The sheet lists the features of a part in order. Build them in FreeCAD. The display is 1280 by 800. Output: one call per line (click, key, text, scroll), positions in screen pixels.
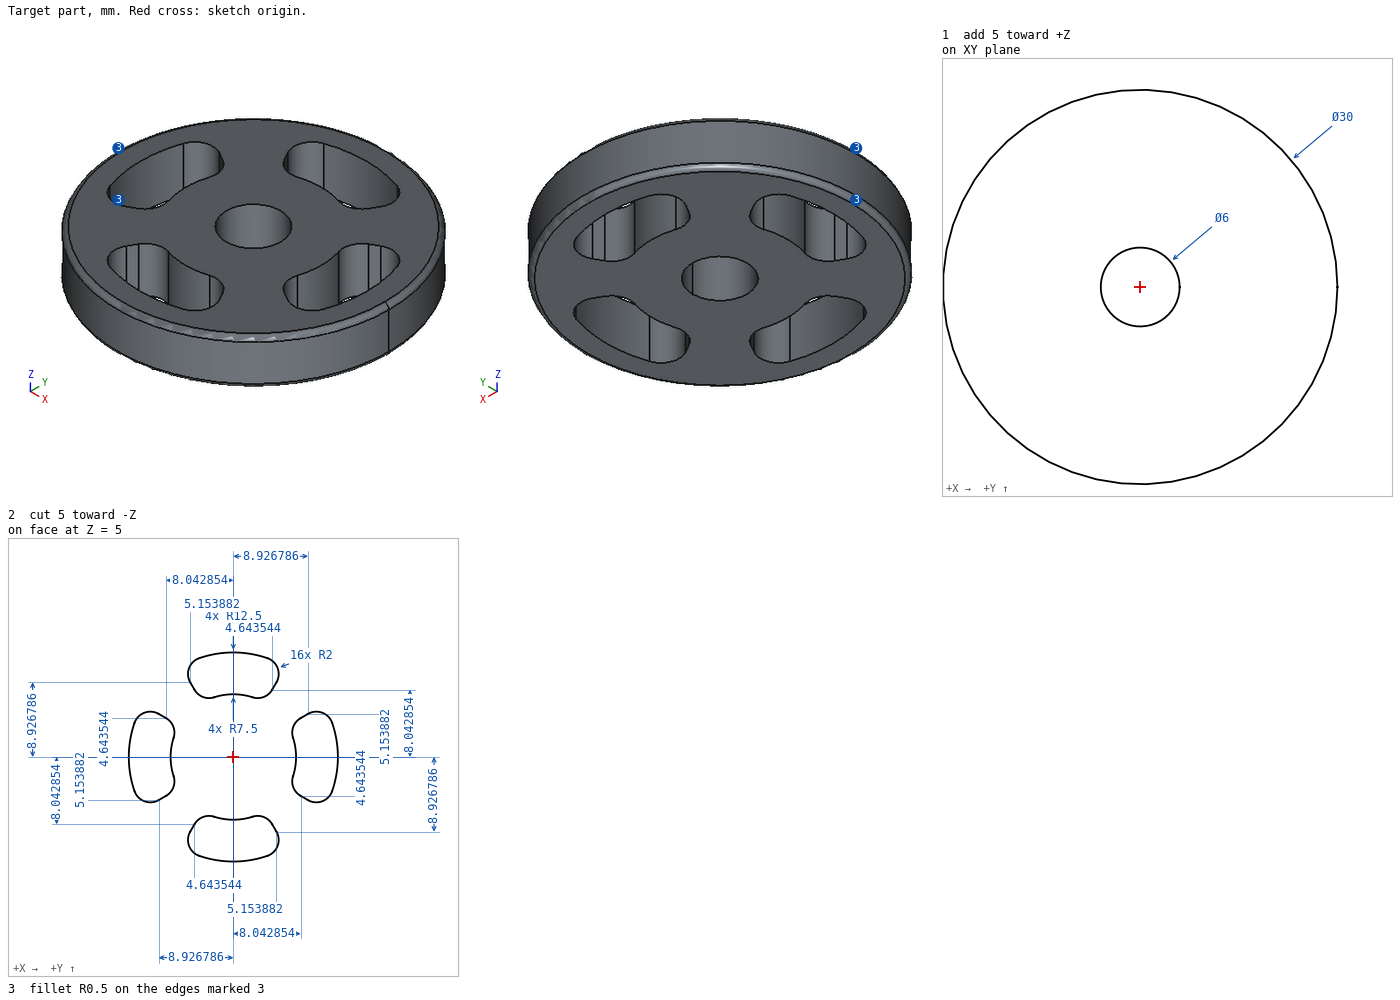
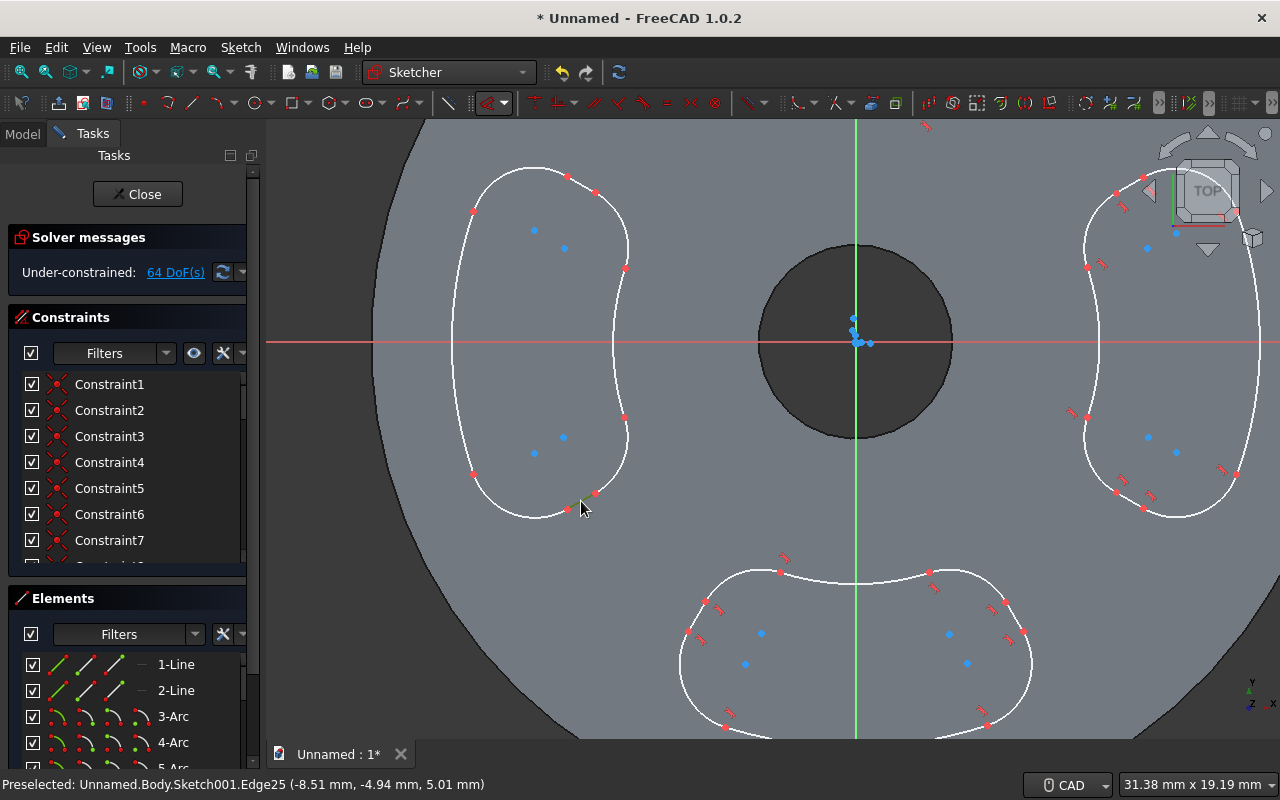
click(615, 476)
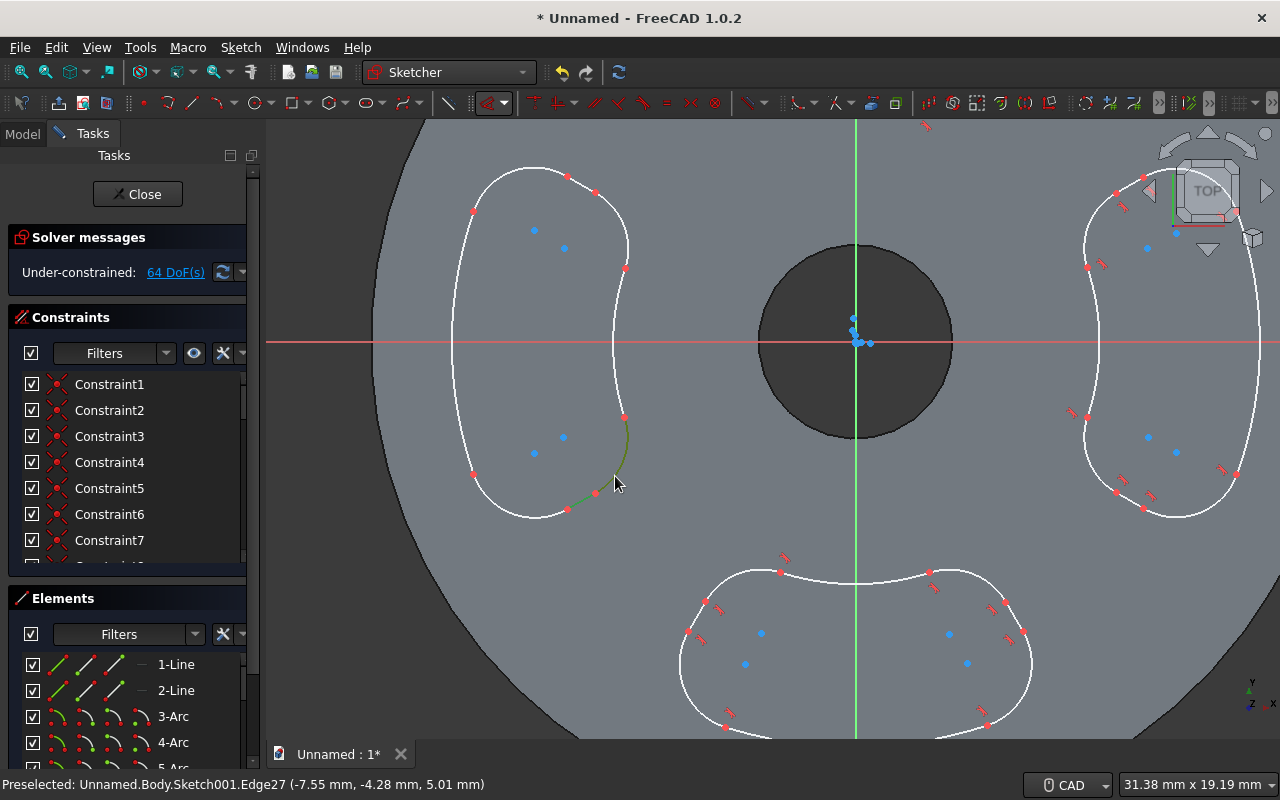
click(644, 104)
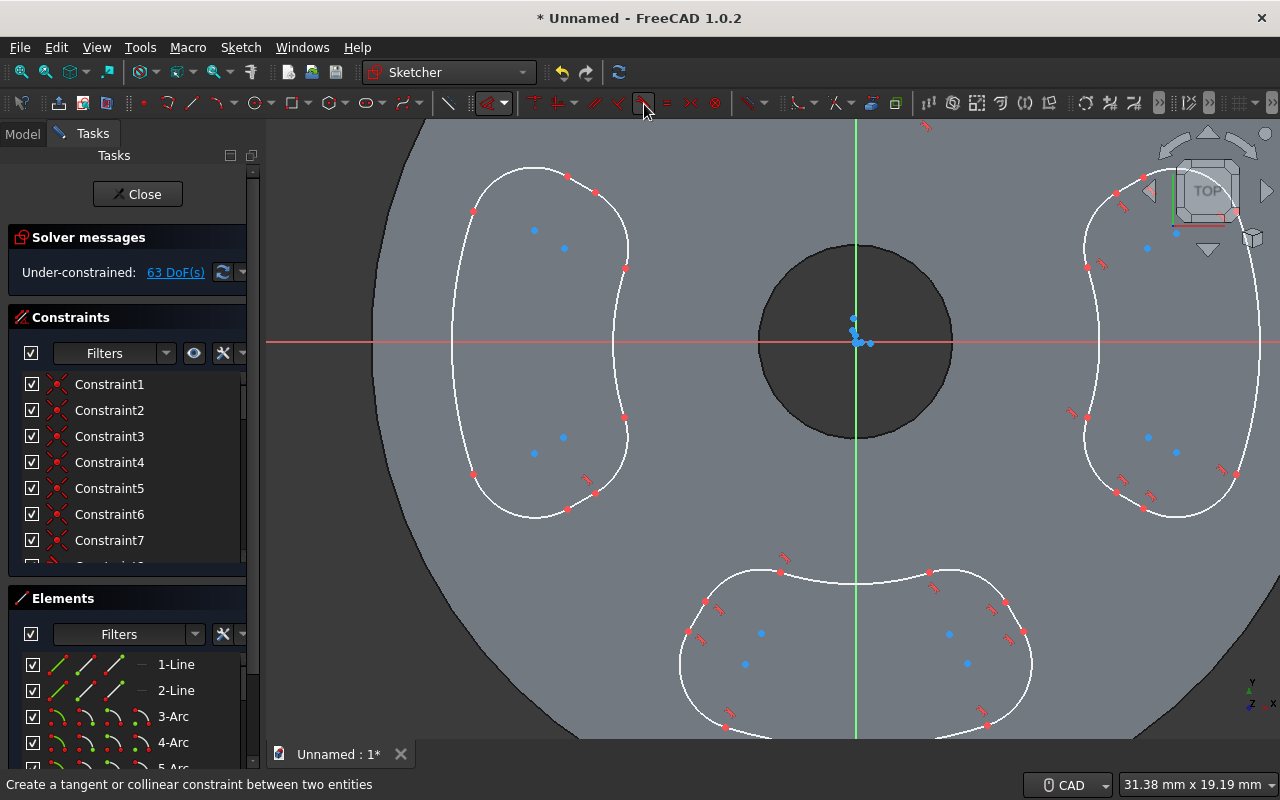
scroll(576, 504, up, 2)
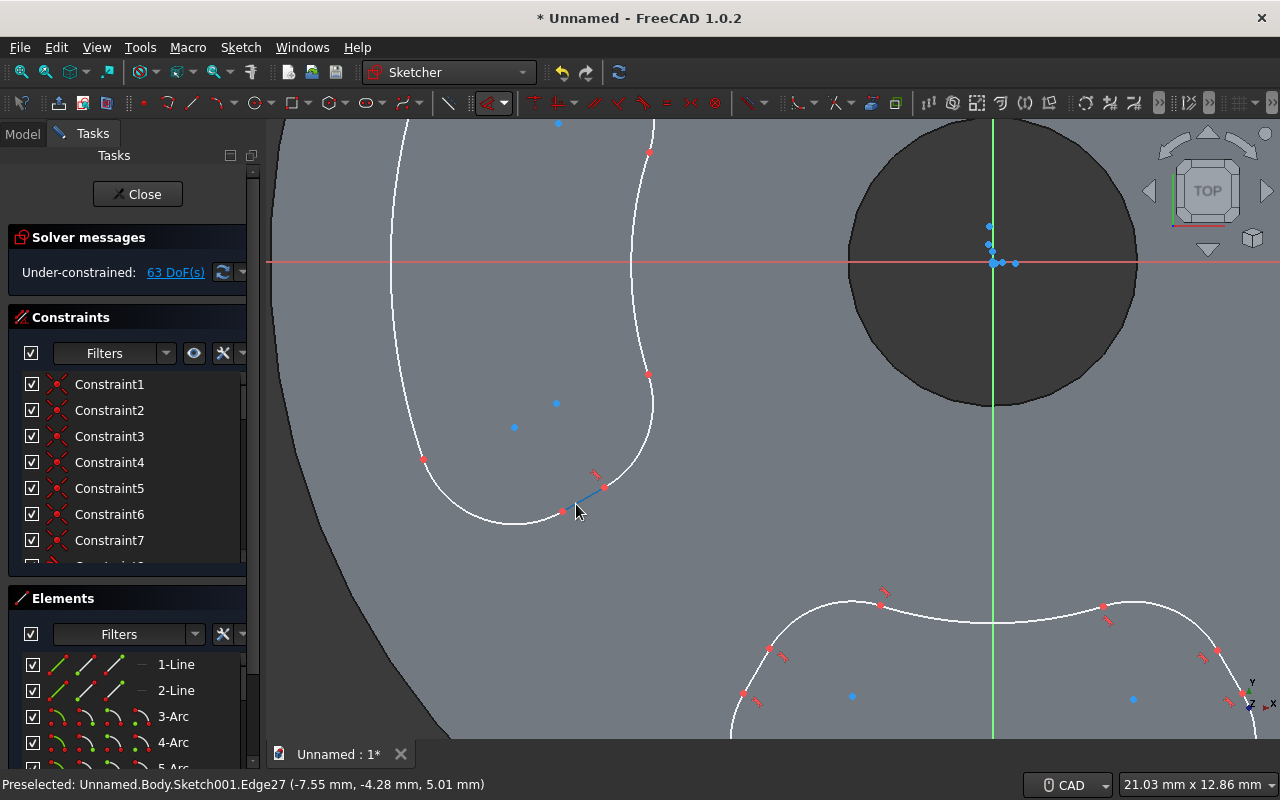
click(575, 504)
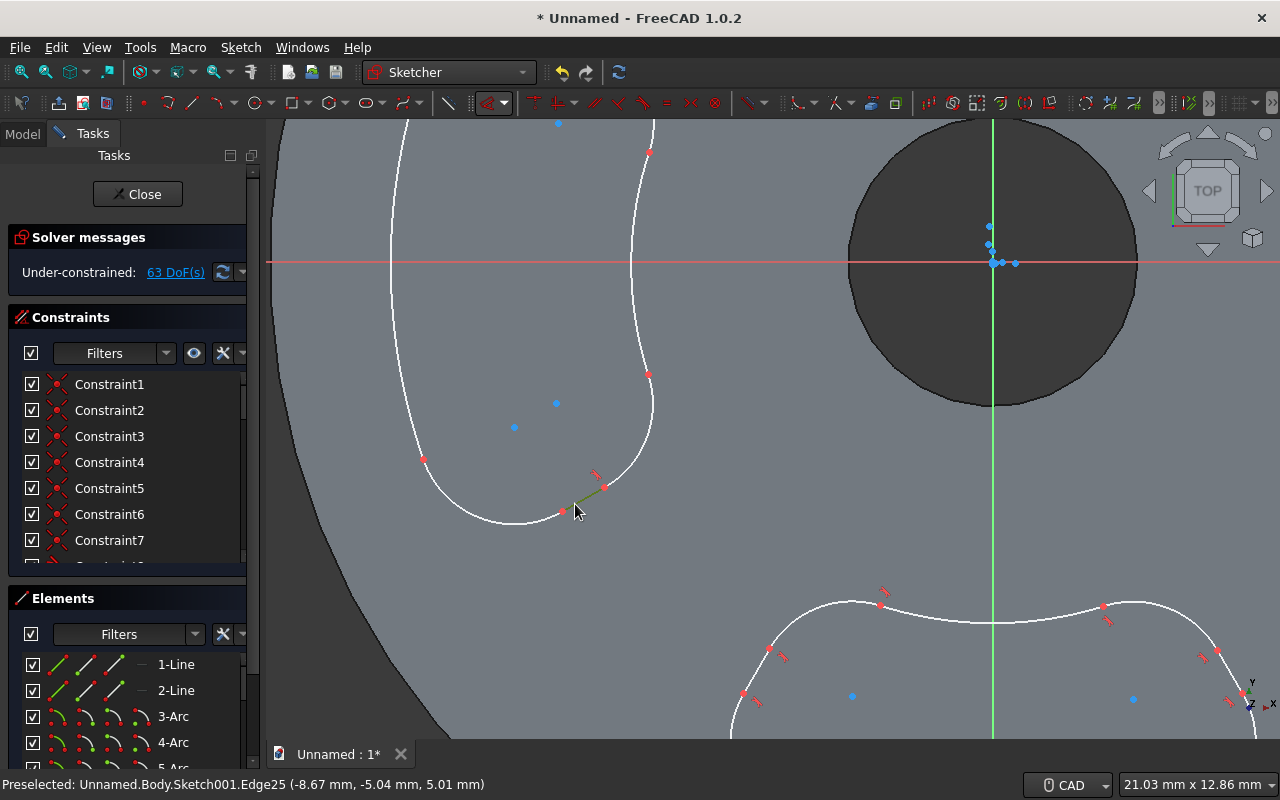
click(452, 501)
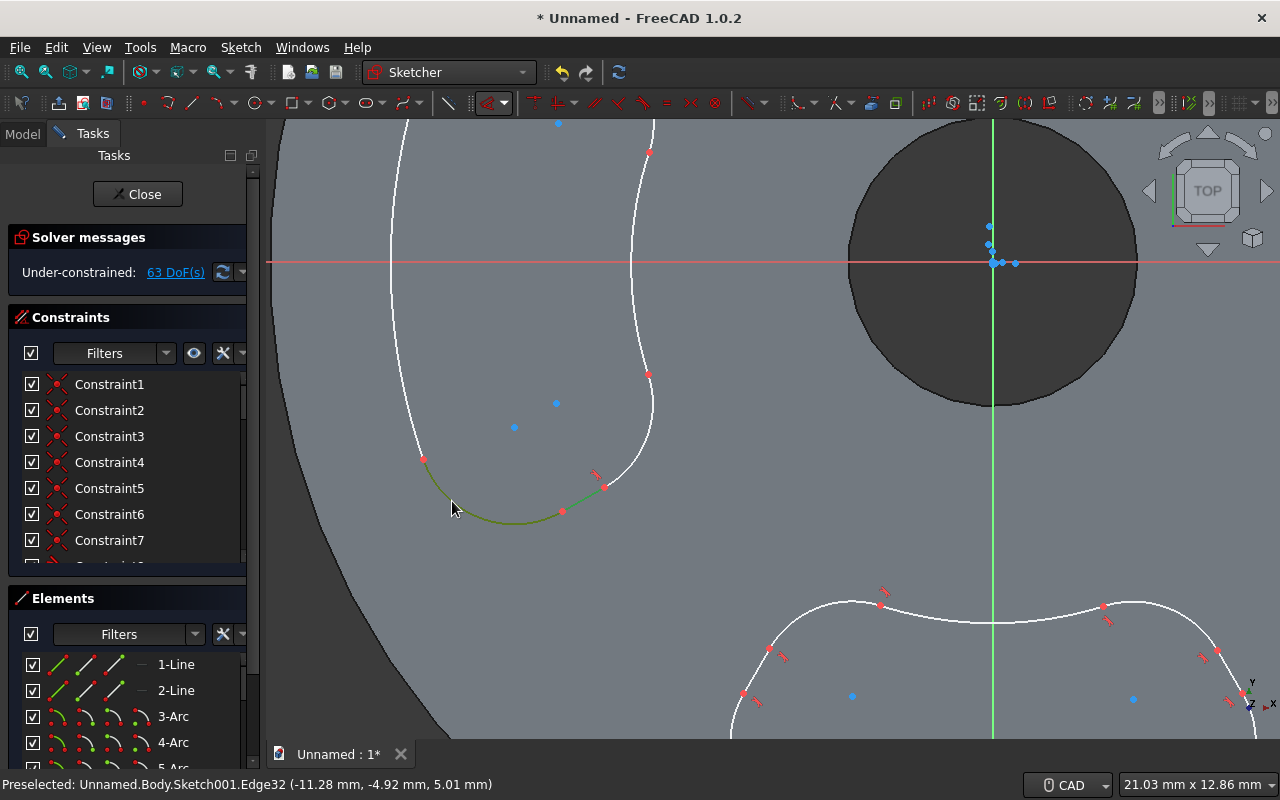
click(644, 104)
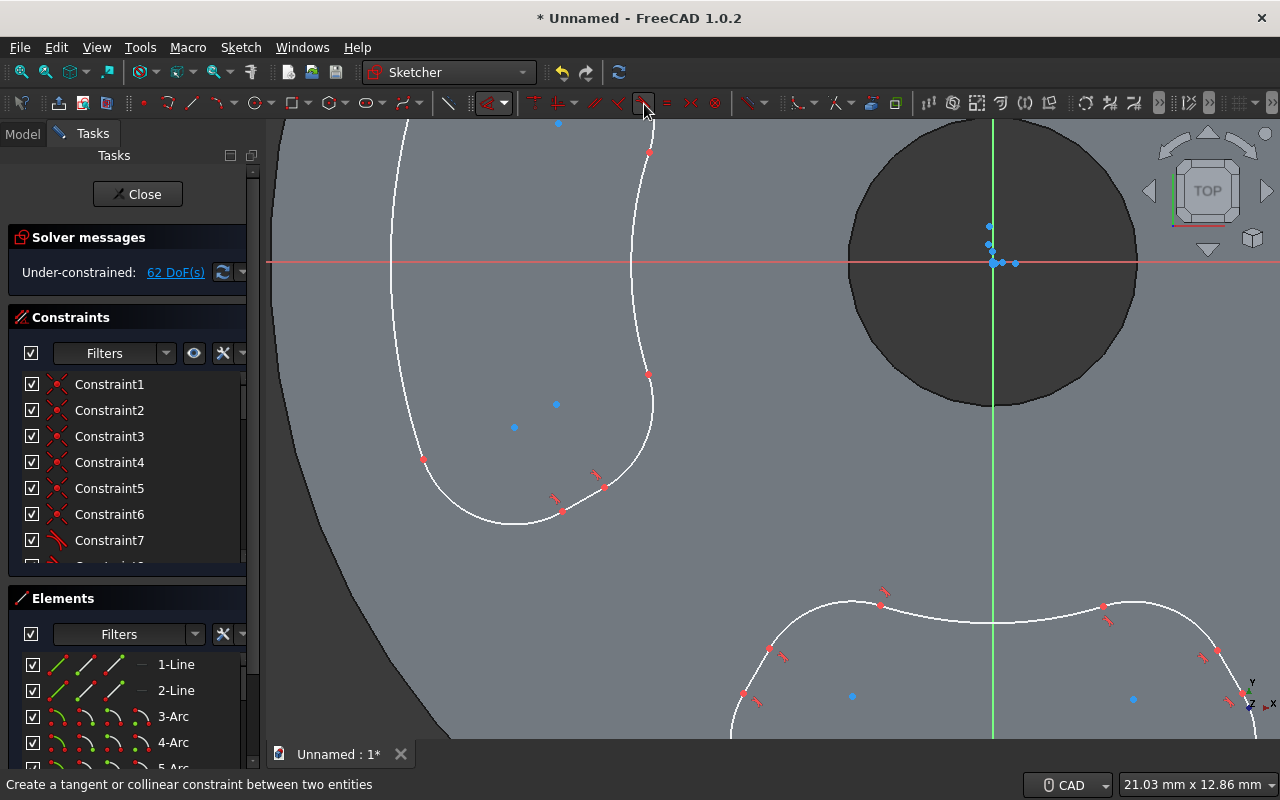
scroll(580, 501, down, 6)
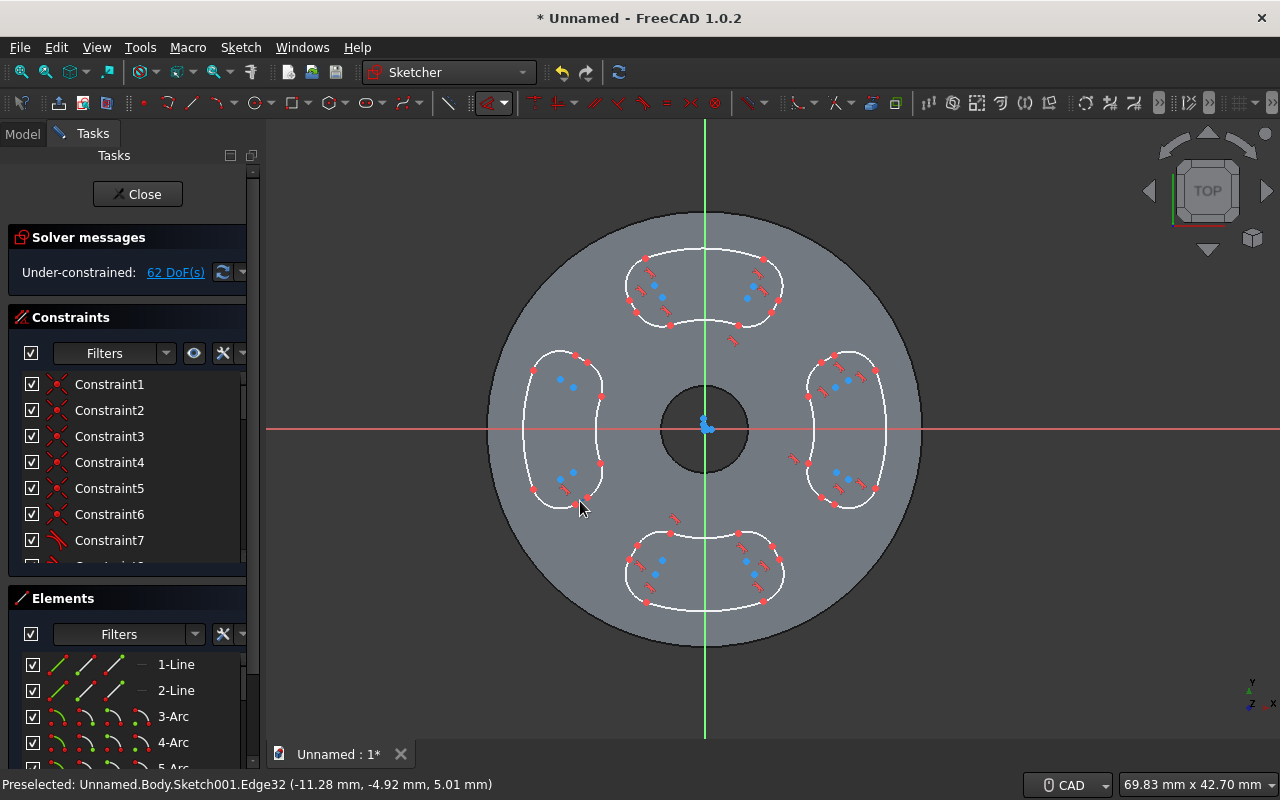
scroll(584, 360, up, 6)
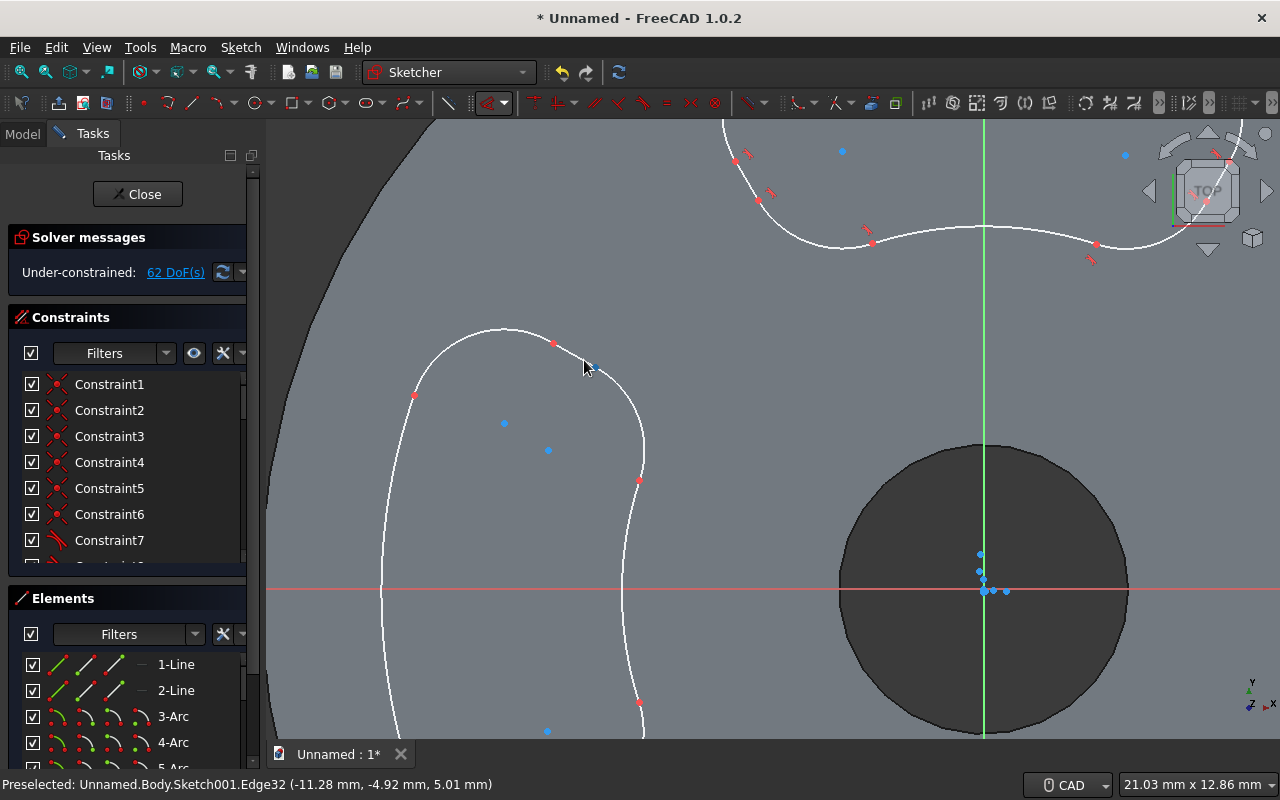
click(583, 360)